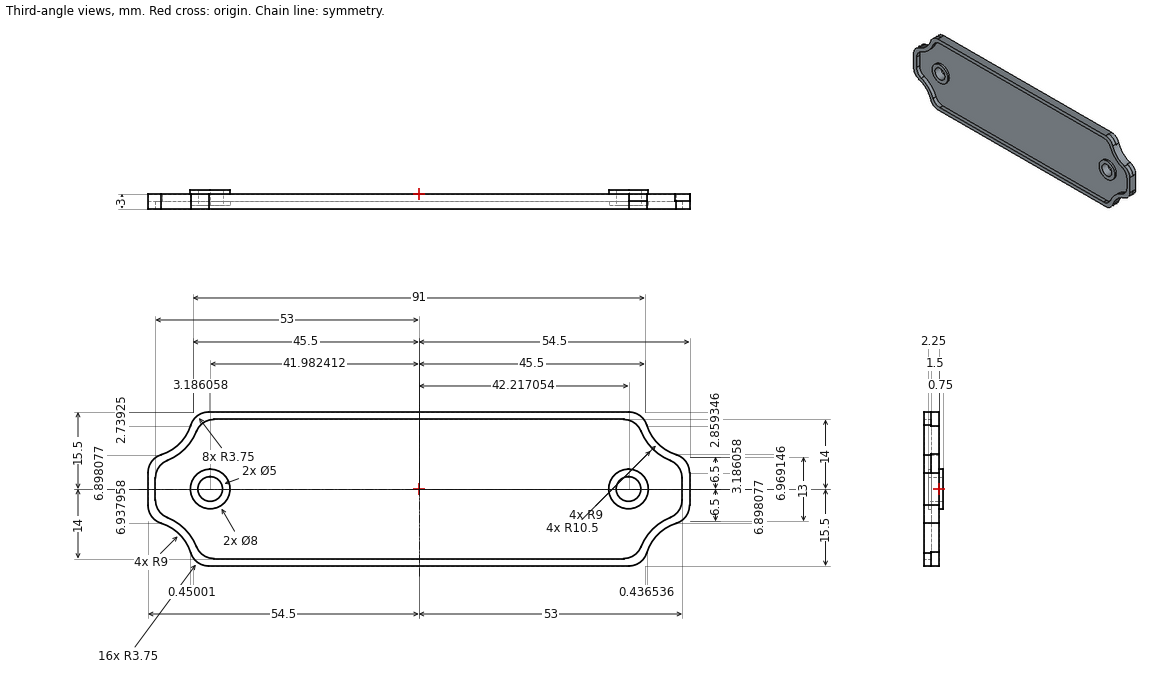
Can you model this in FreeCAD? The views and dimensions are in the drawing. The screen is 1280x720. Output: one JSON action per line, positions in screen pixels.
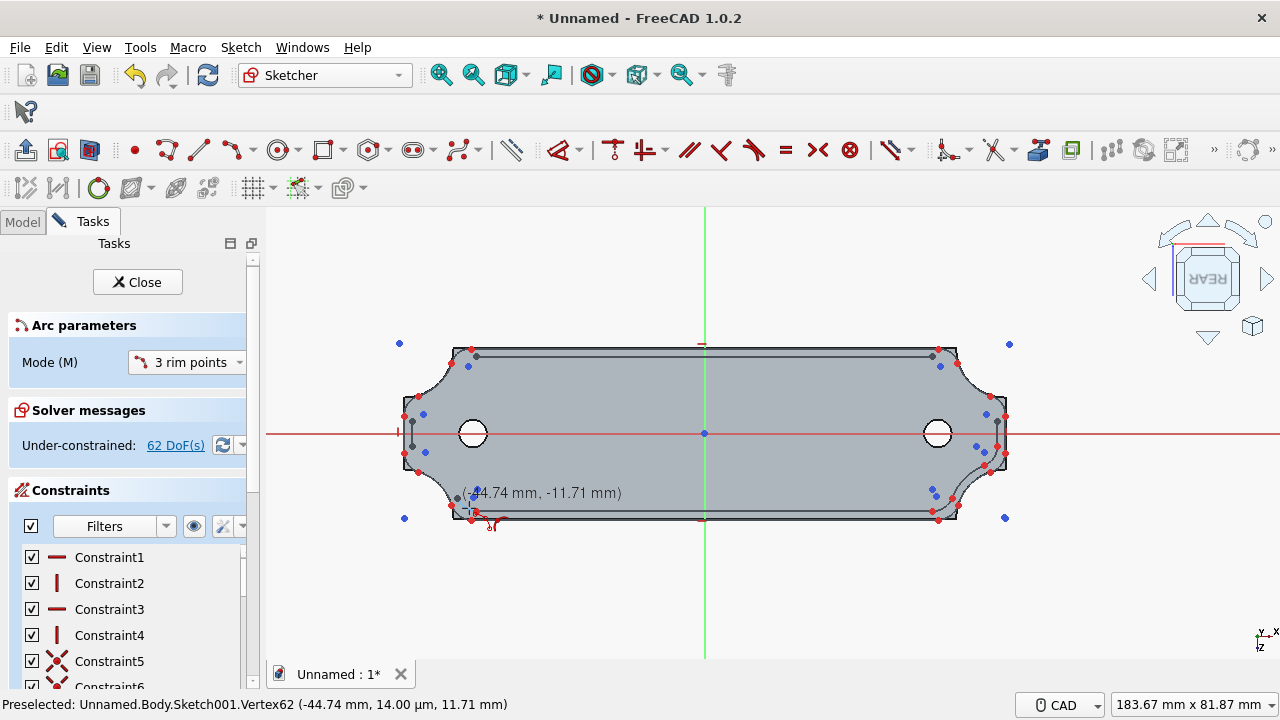
{"action": "scroll", "coordinate": [425, 465], "scroll_direction": "up", "scroll_amount": 4}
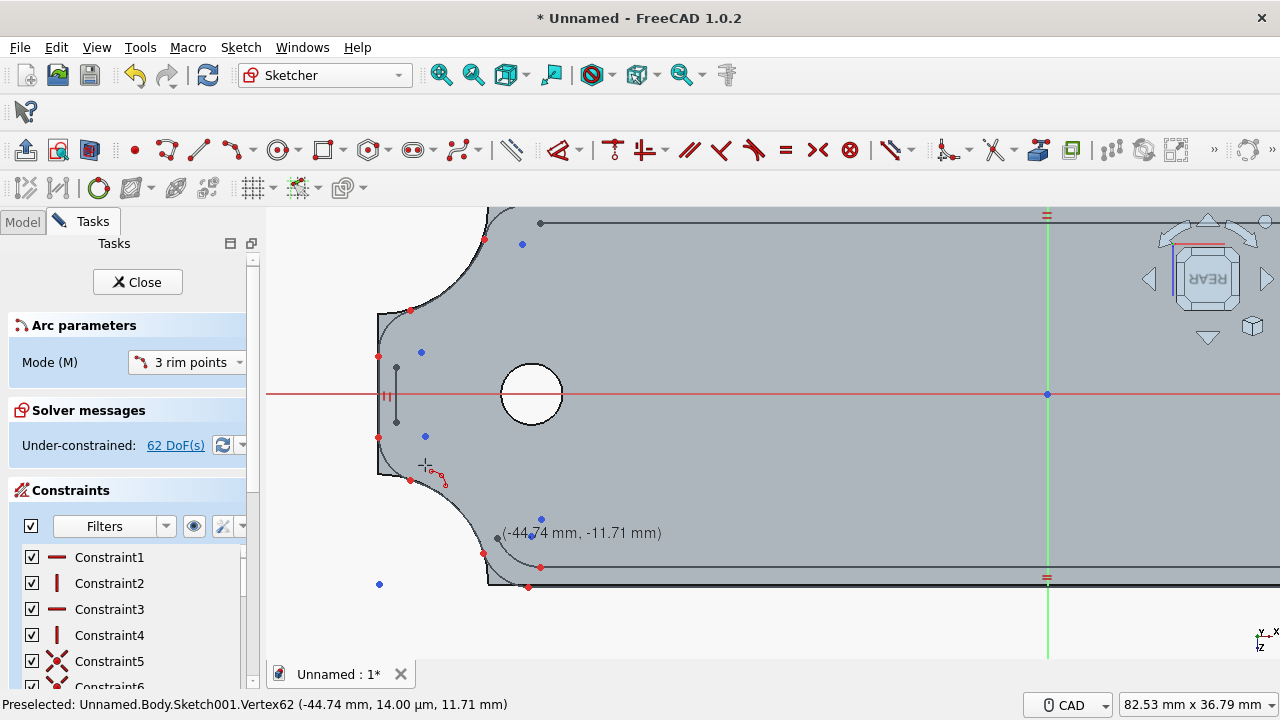
{"action": "left_click", "coordinate": [425, 465]}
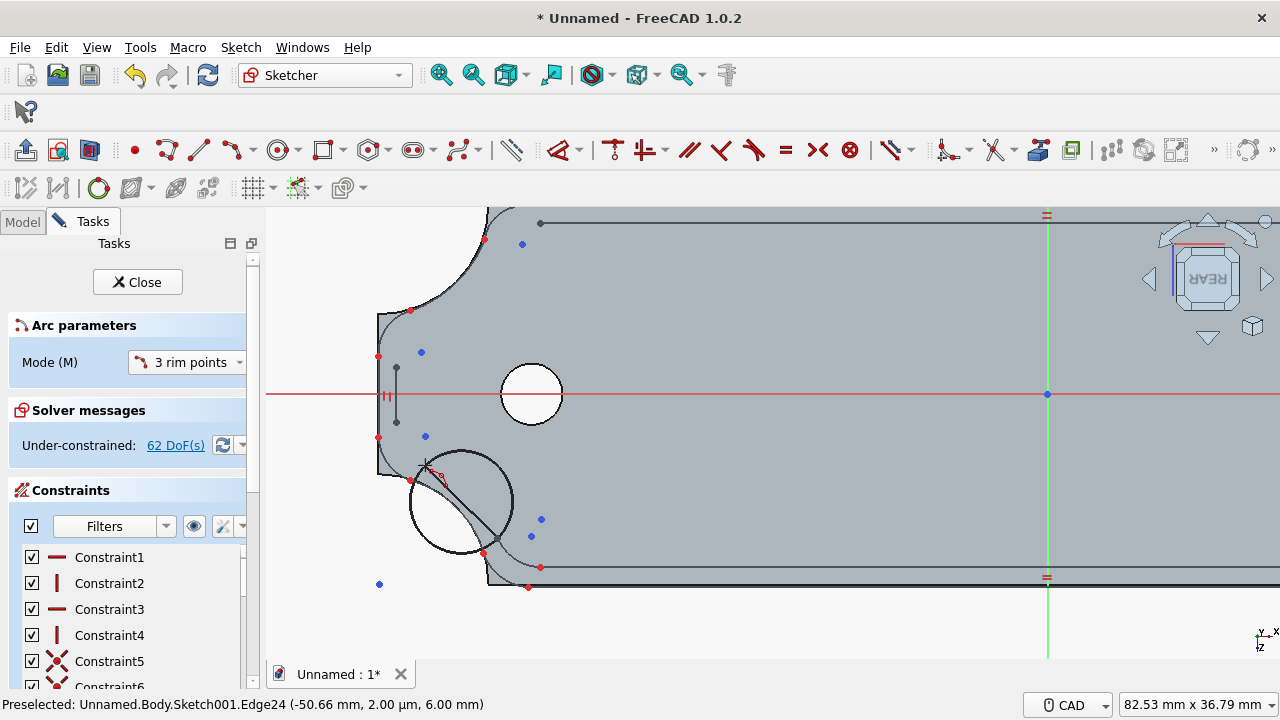
{"action": "scroll", "coordinate": [469, 493], "scroll_direction": "up", "scroll_amount": 3}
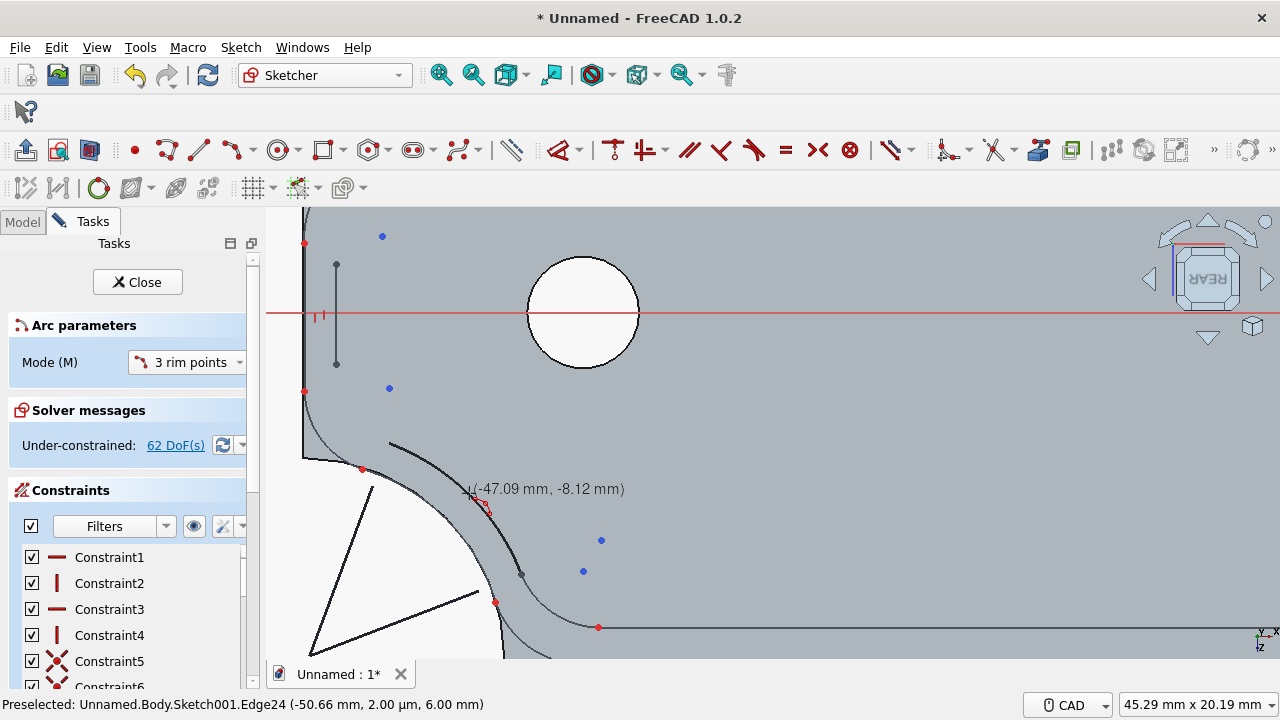
{"action": "left_click", "coordinate": [469, 493]}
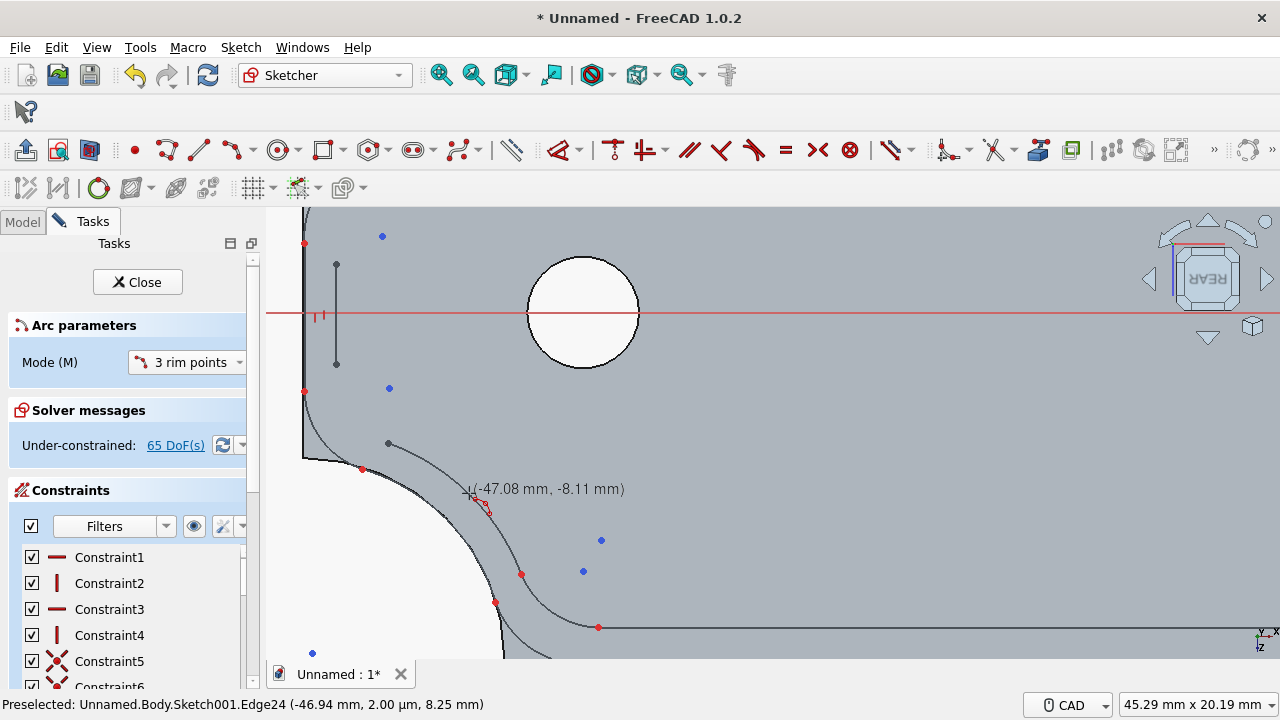
{"action": "left_click", "coordinate": [389, 443]}
{"action": "left_click", "coordinate": [336, 364]}
{"action": "left_click", "coordinate": [351, 410]}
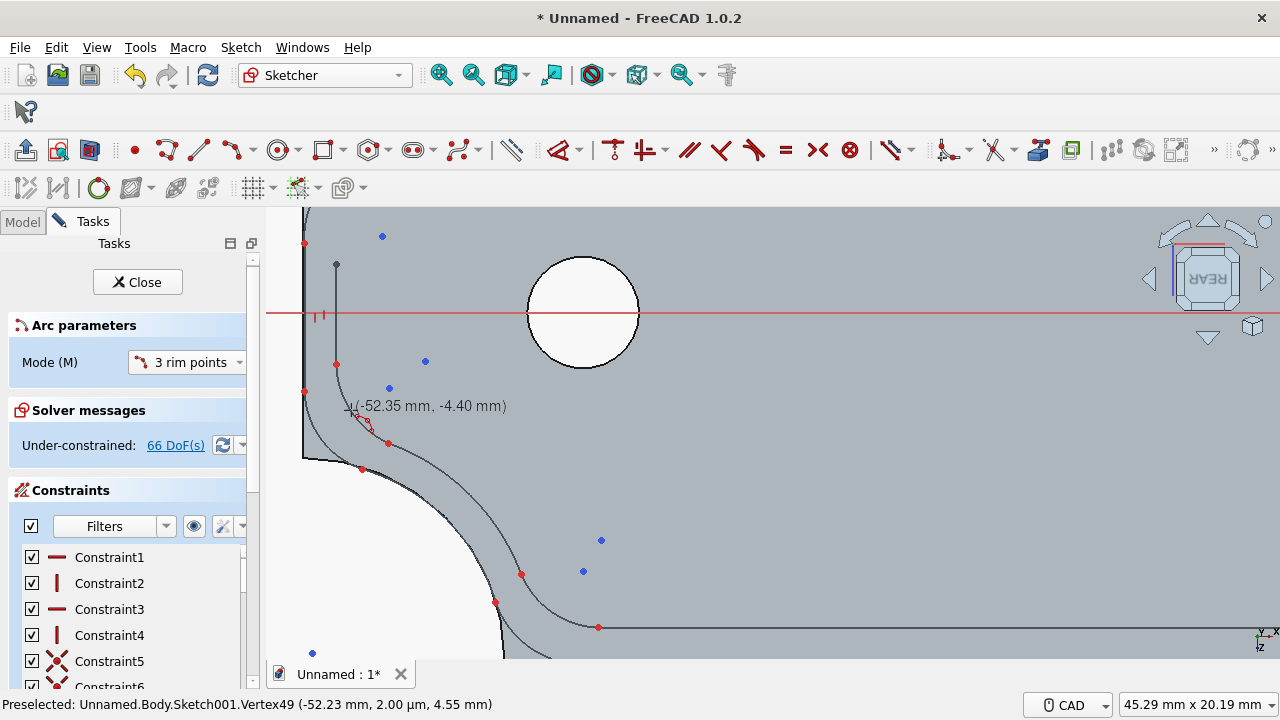
{"action": "left_click", "coordinate": [336, 264]}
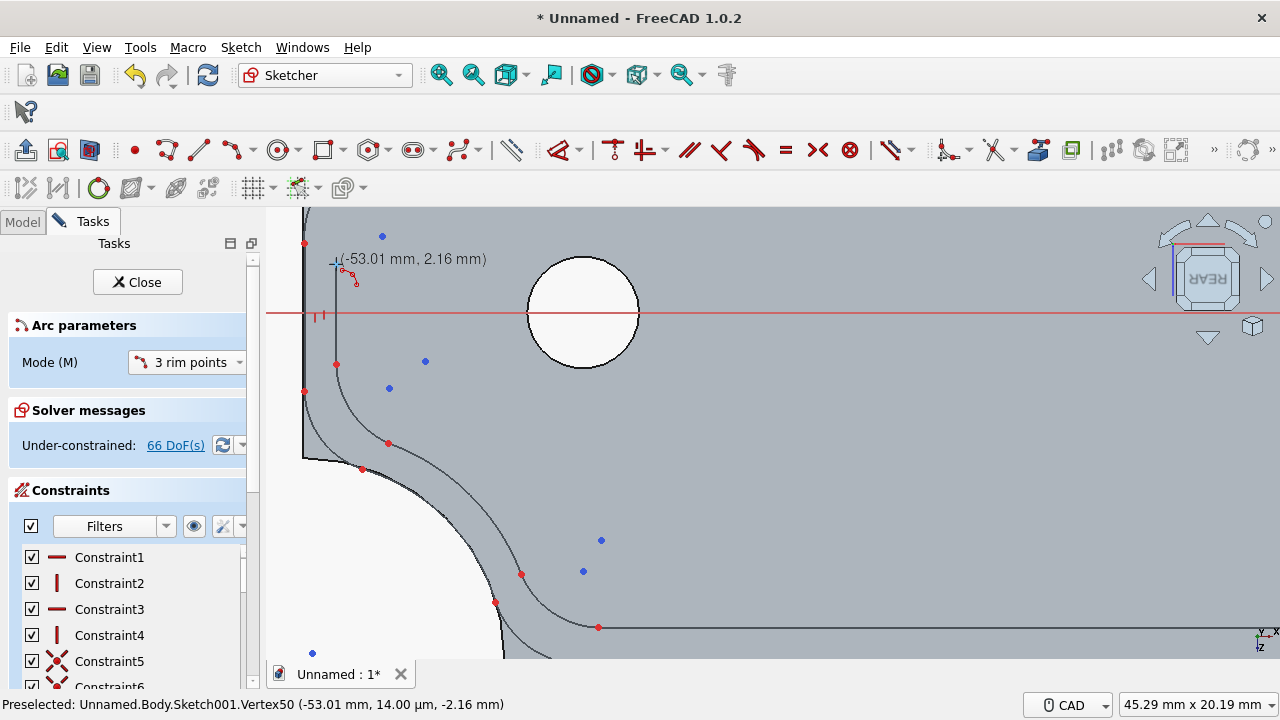
{"action": "scroll", "coordinate": [437, 472], "scroll_direction": "down", "scroll_amount": 7}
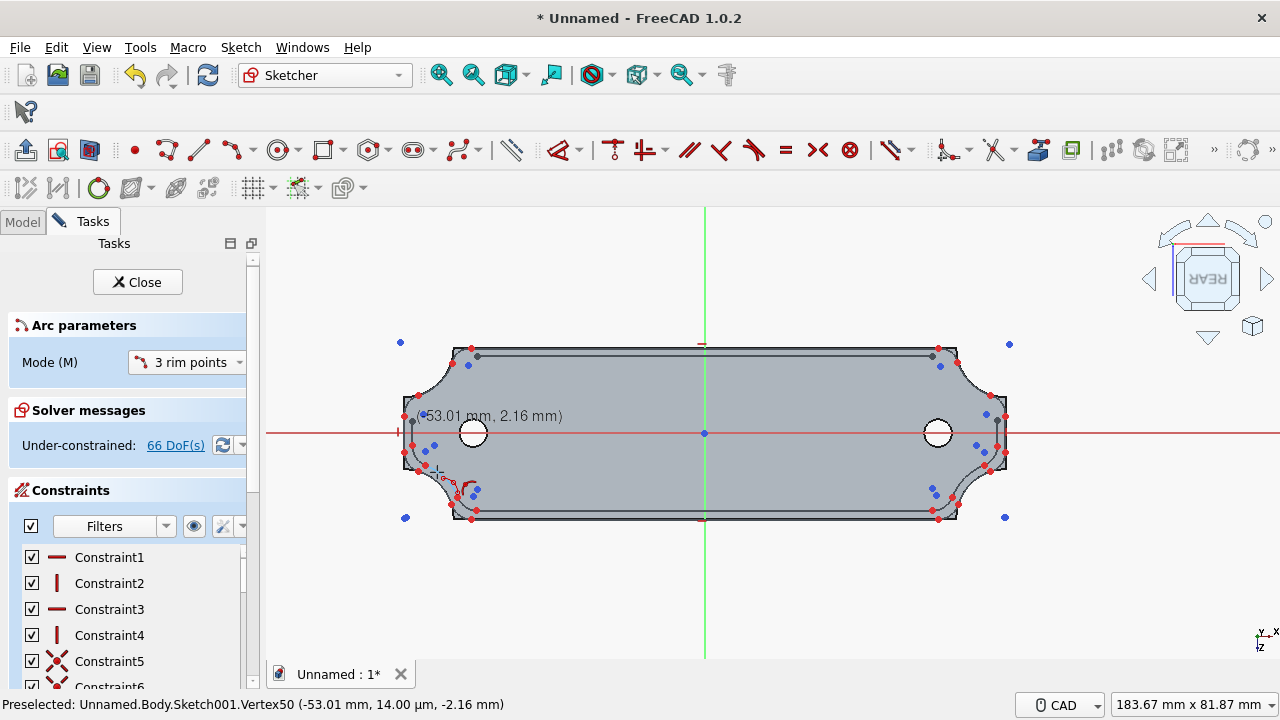
{"action": "scroll", "coordinate": [425, 401], "scroll_direction": "up", "scroll_amount": 4}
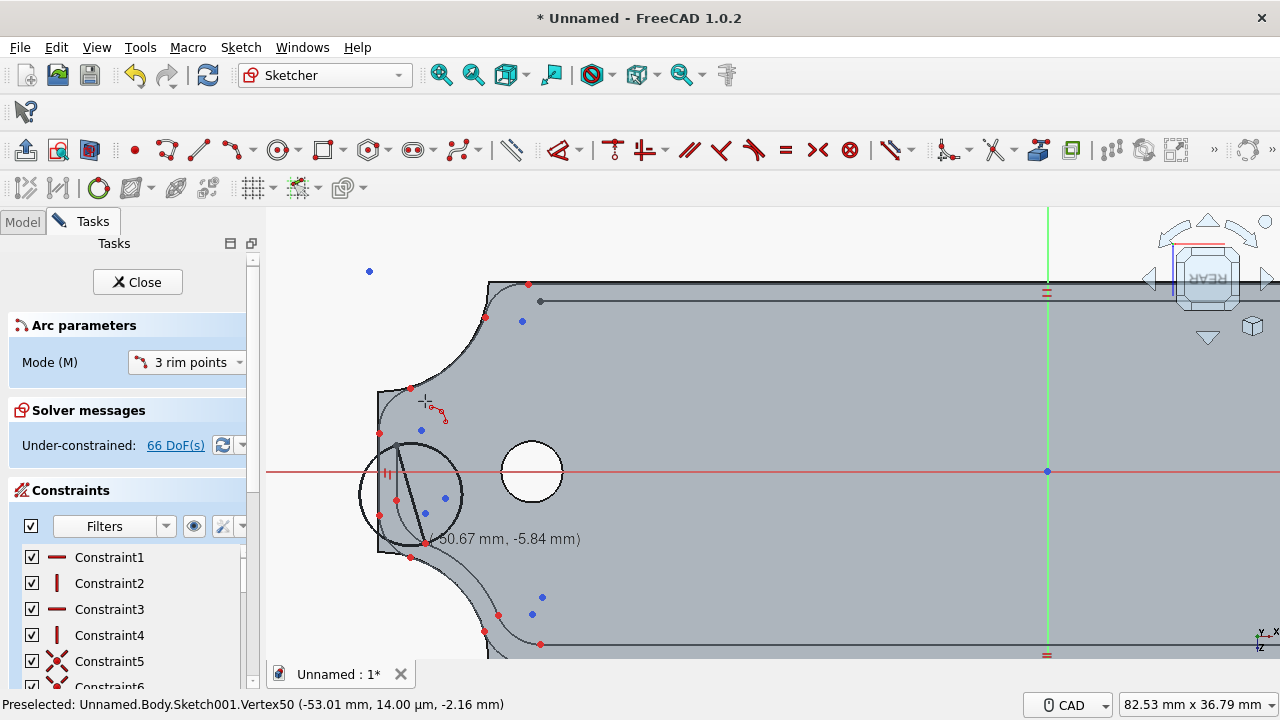
{"action": "left_click", "coordinate": [426, 401]}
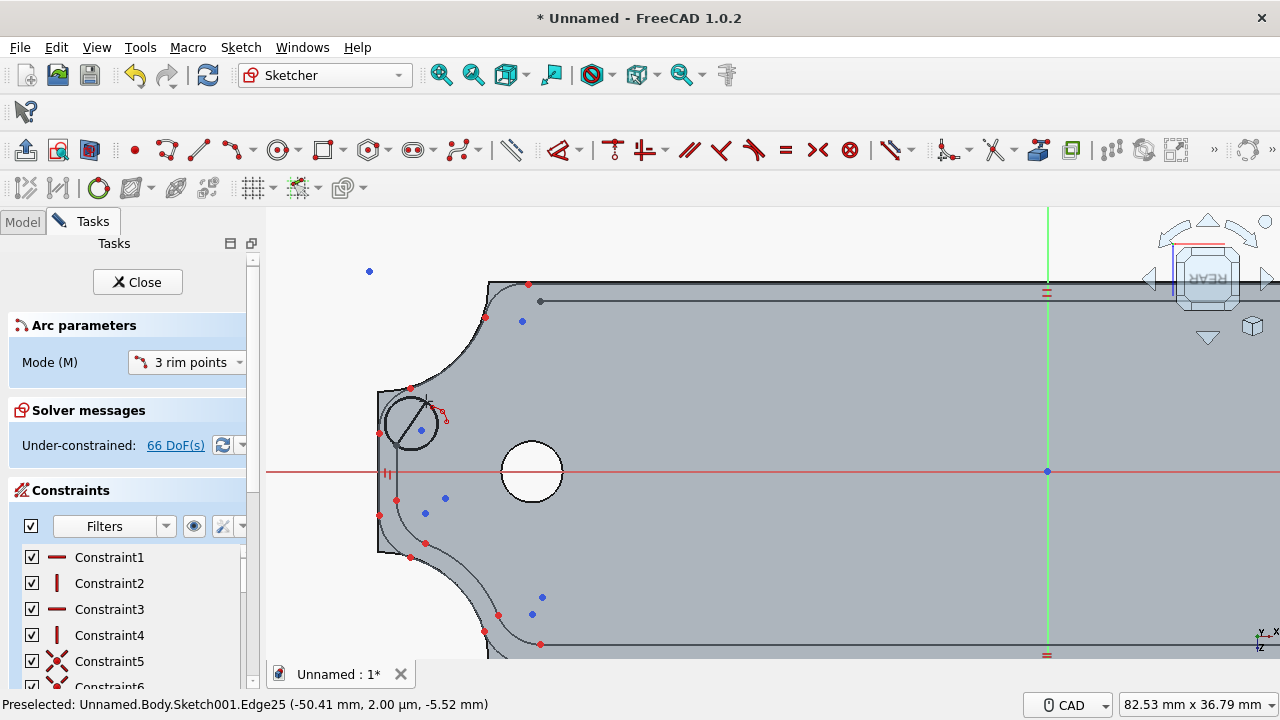
{"action": "scroll", "coordinate": [405, 418], "scroll_direction": "up", "scroll_amount": 4}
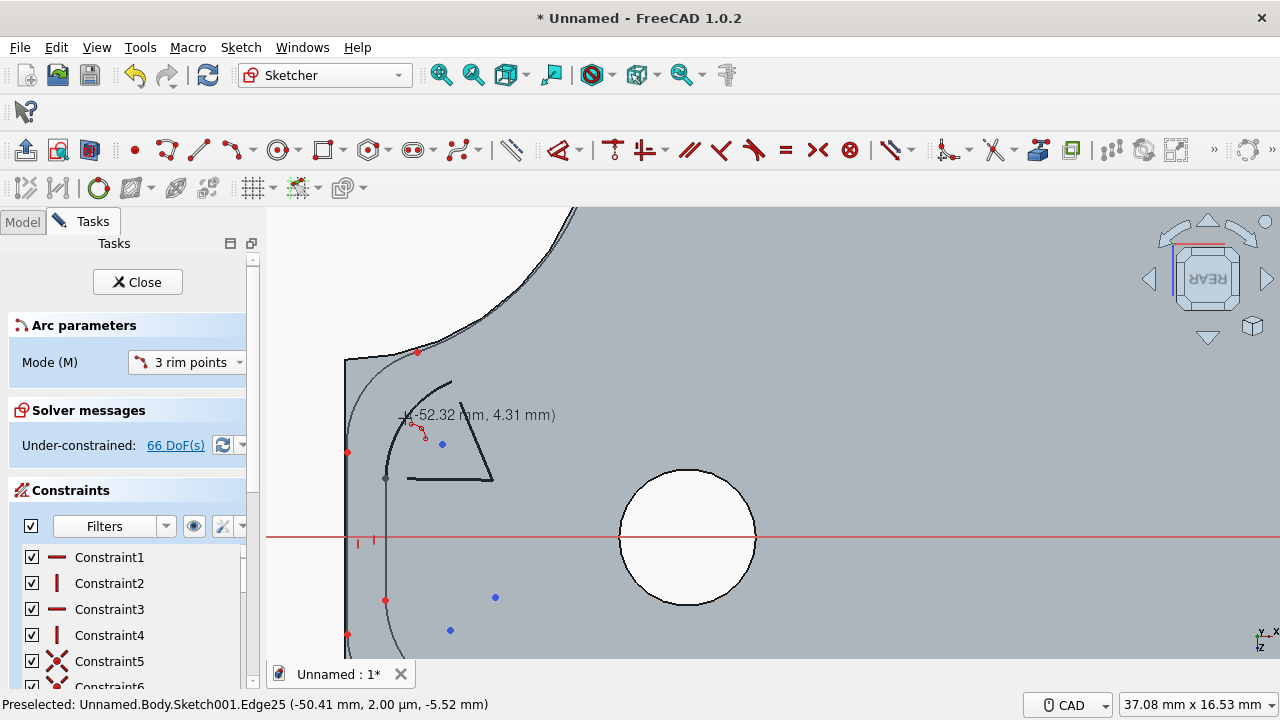
{"action": "left_click", "coordinate": [404, 418]}